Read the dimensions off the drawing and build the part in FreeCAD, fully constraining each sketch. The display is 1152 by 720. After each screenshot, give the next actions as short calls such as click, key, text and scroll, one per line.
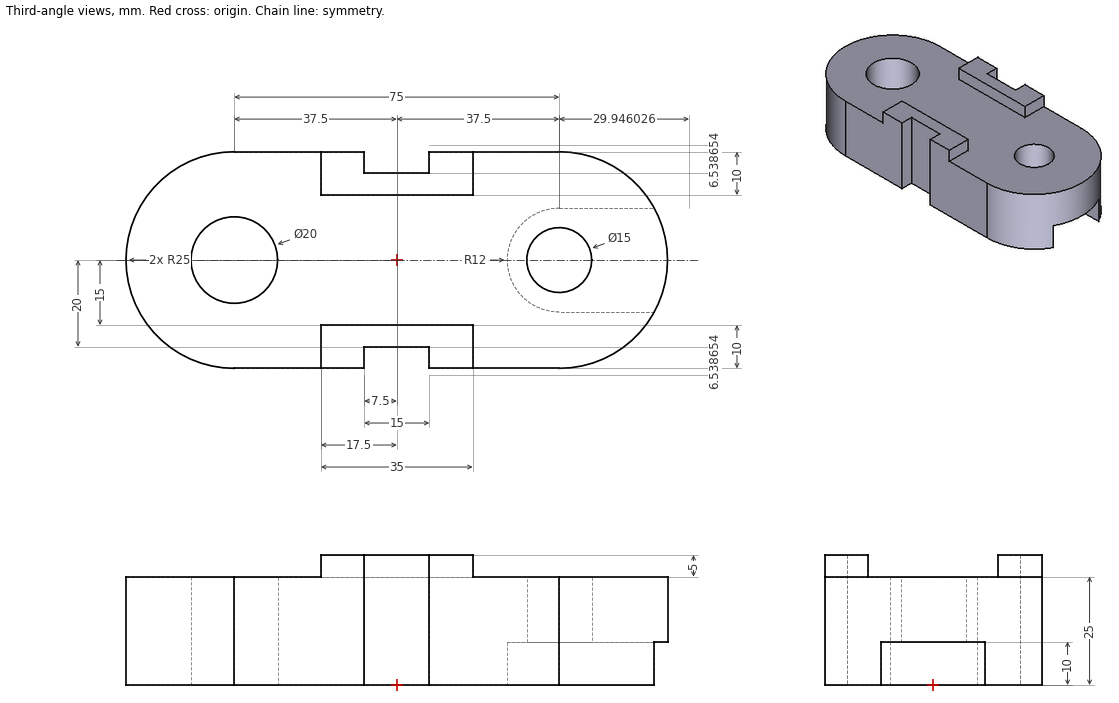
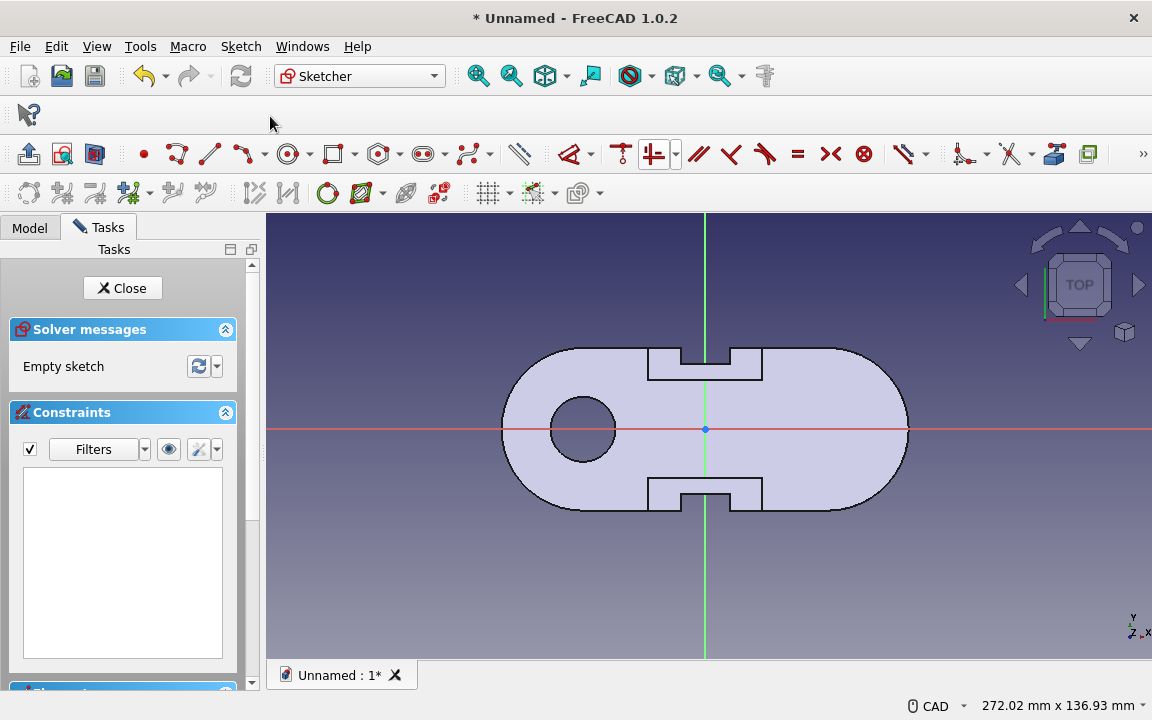
key(q)
key(s)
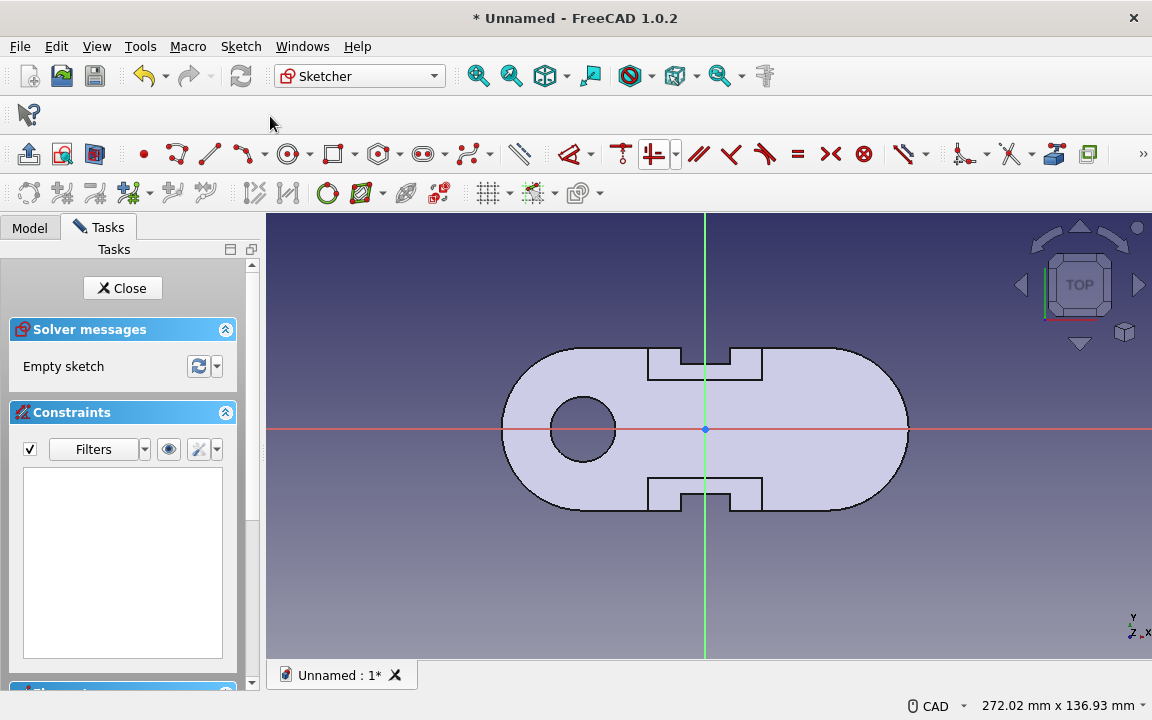
scroll(864, 428, up, 9)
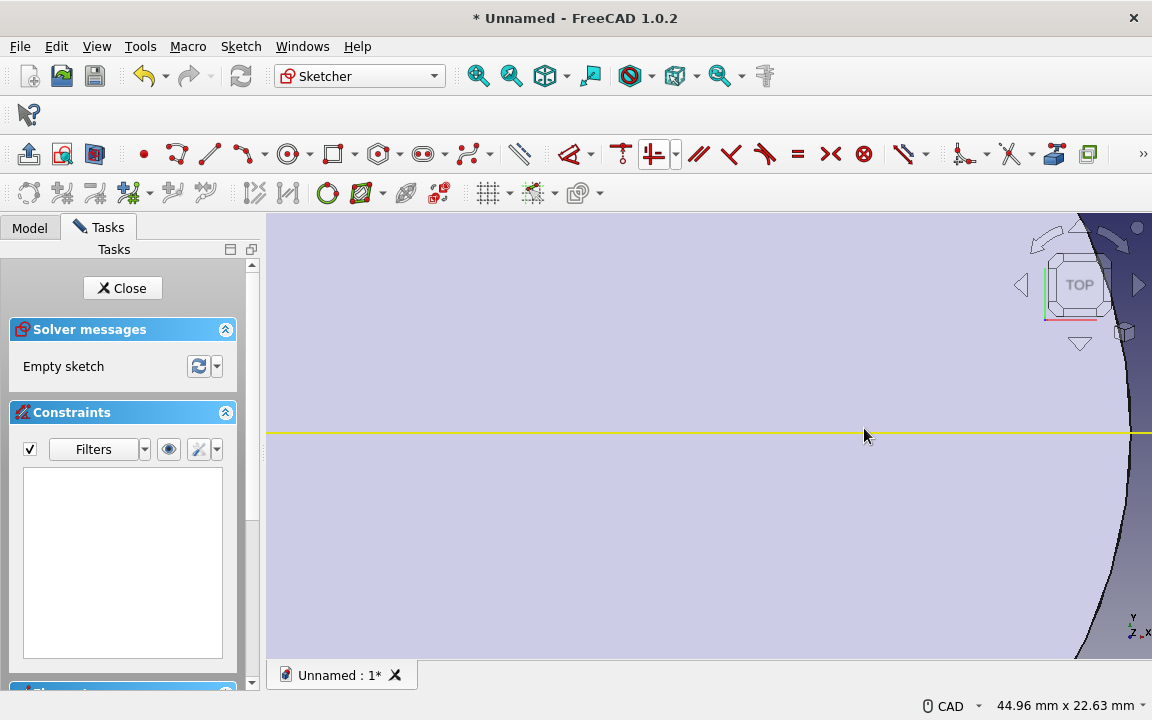
click(288, 154)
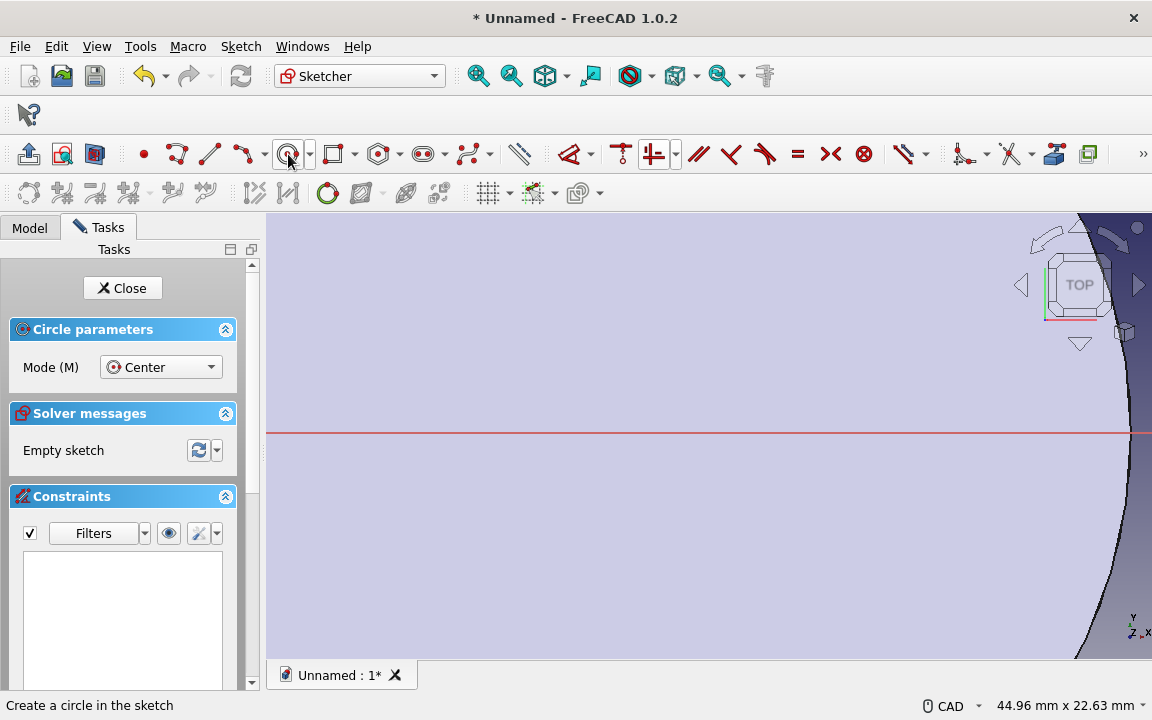
click(638, 433)
move(743, 329)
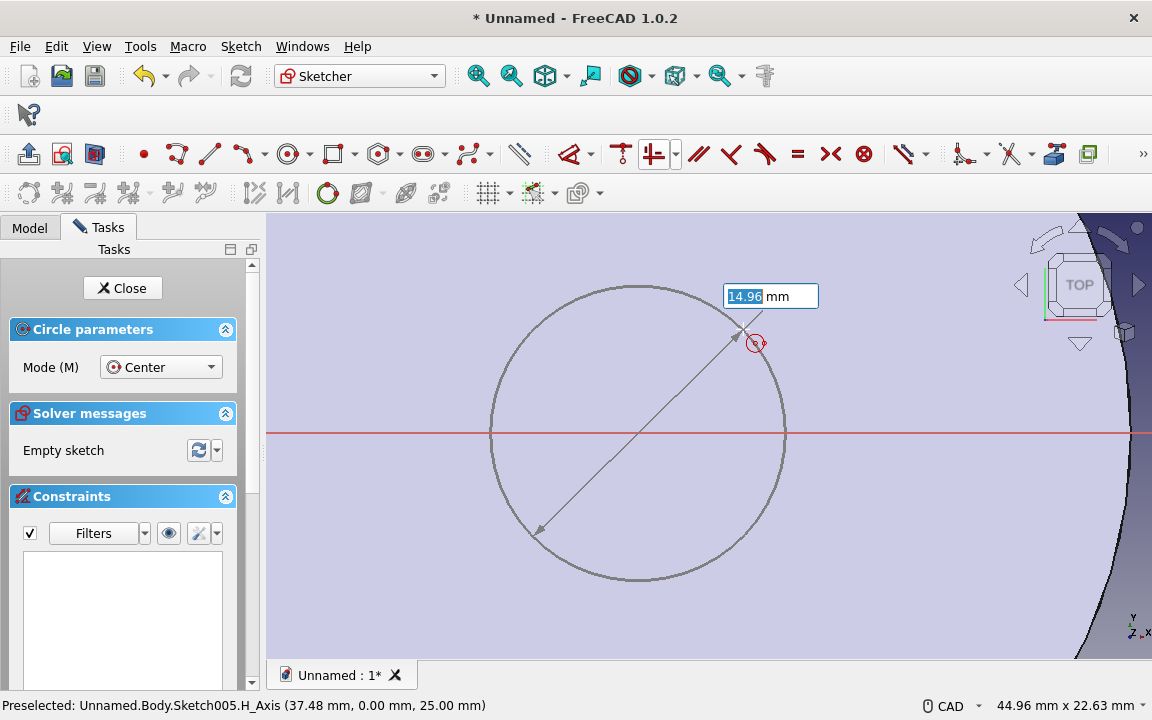
text(15)
key(Return)
key(Escape)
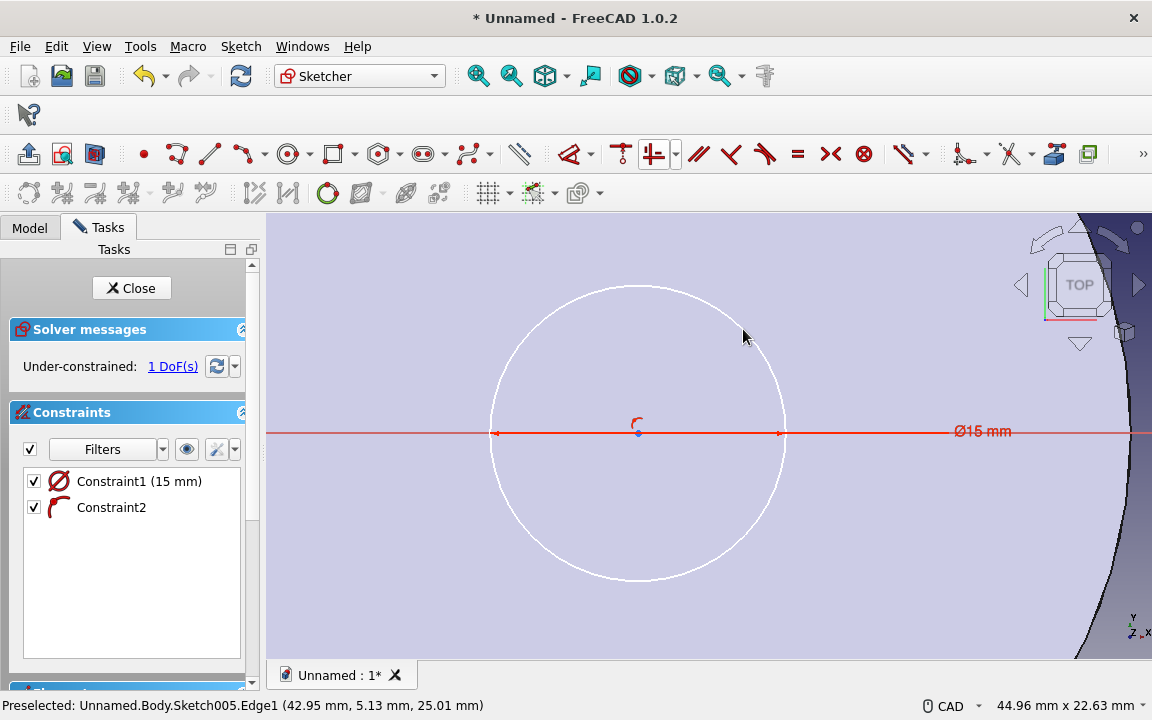
click(568, 154)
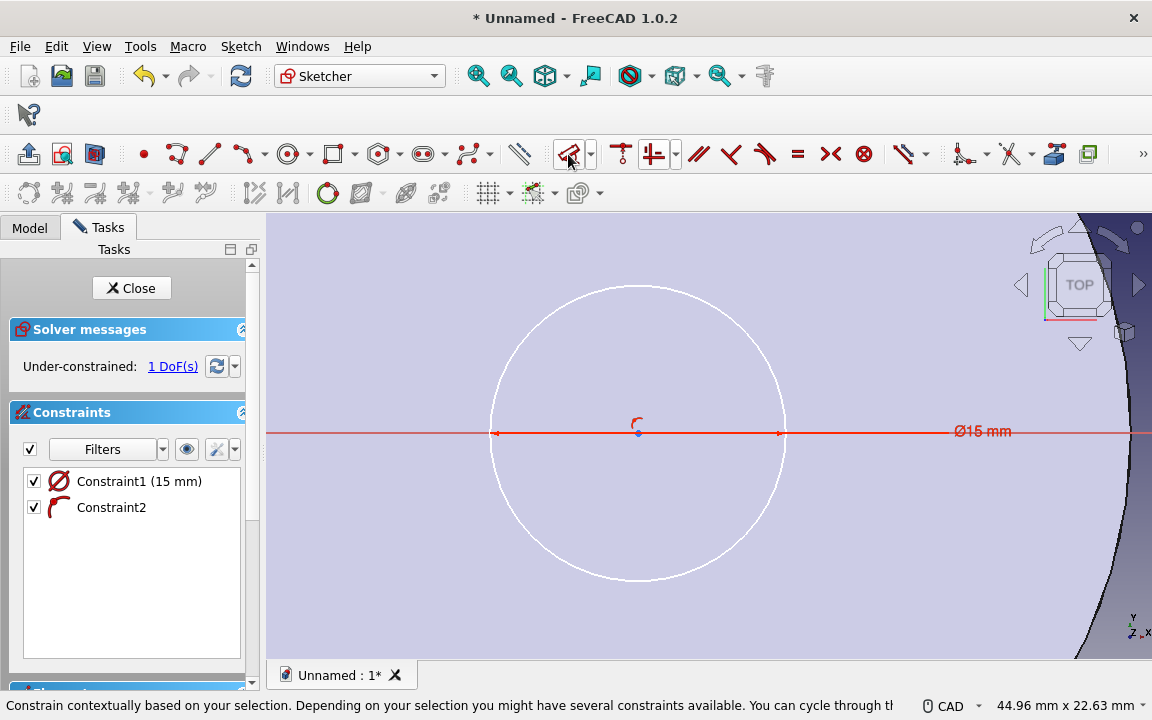
click(638, 433)
click(466, 467)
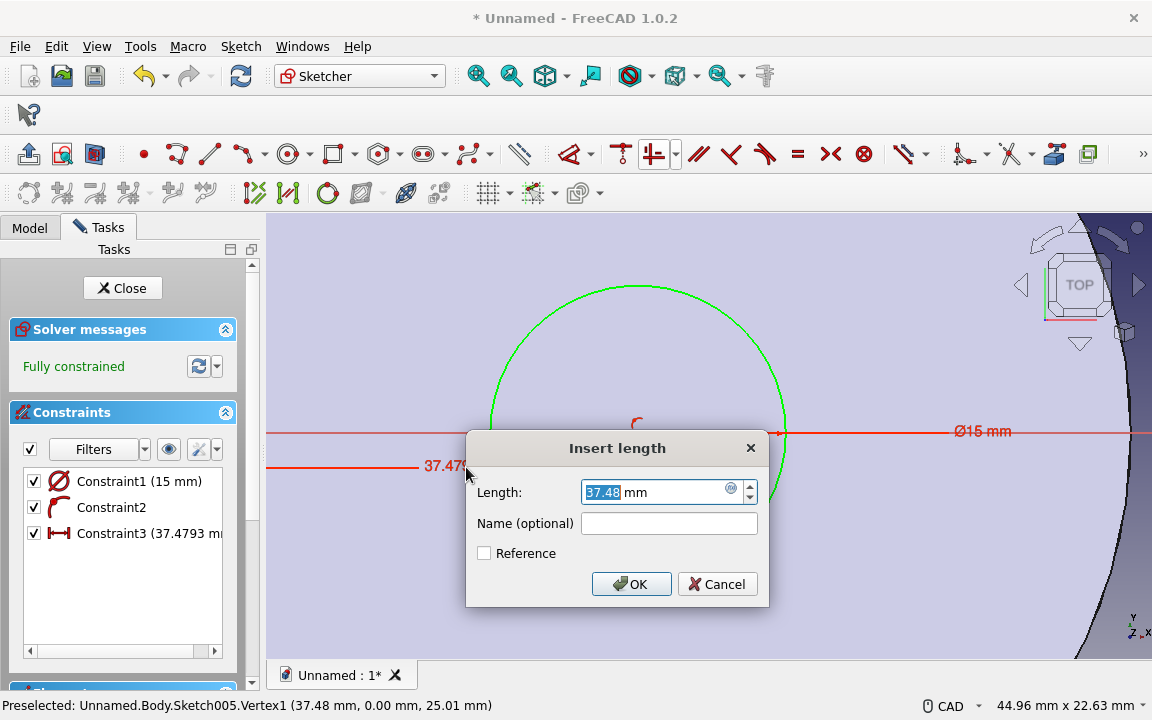
text(37.5)
key(Return)
key(Escape)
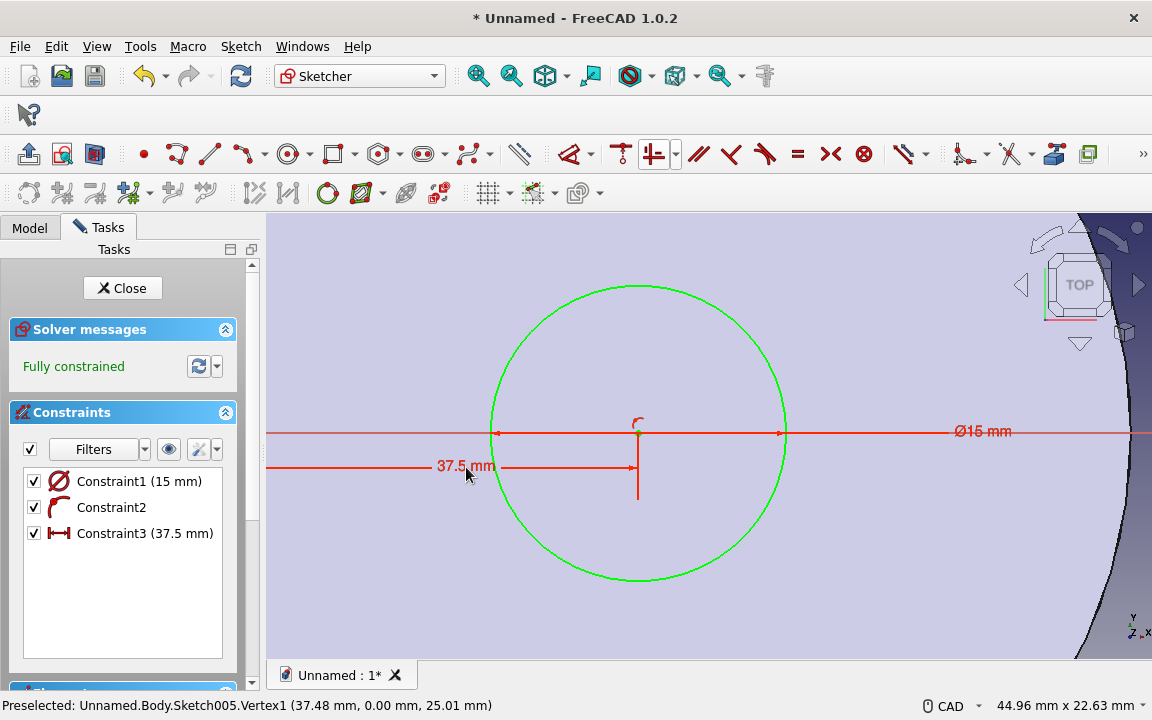
click(123, 288)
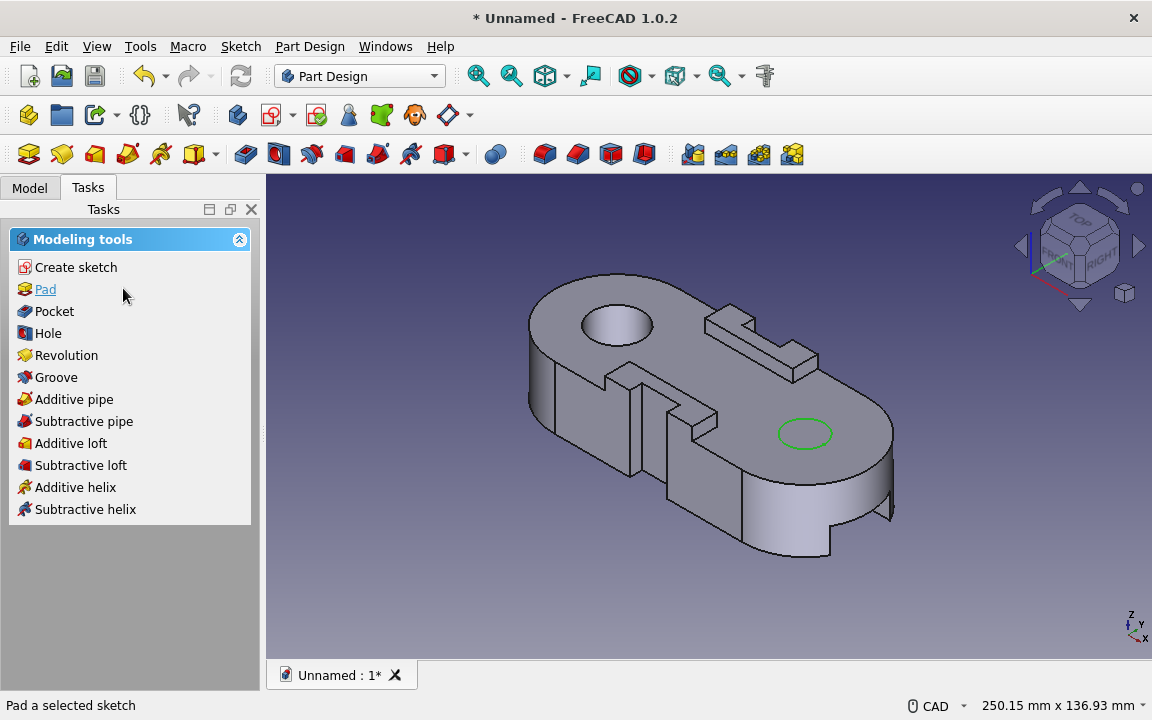
click(246, 154)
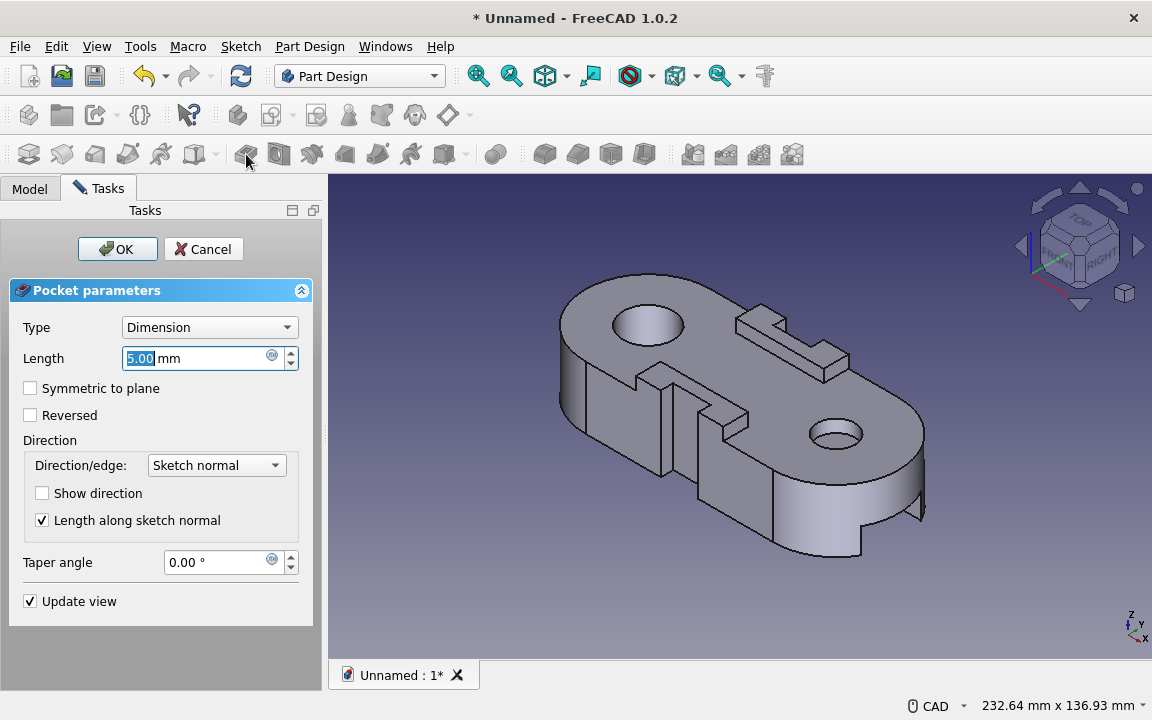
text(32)
key(Tab)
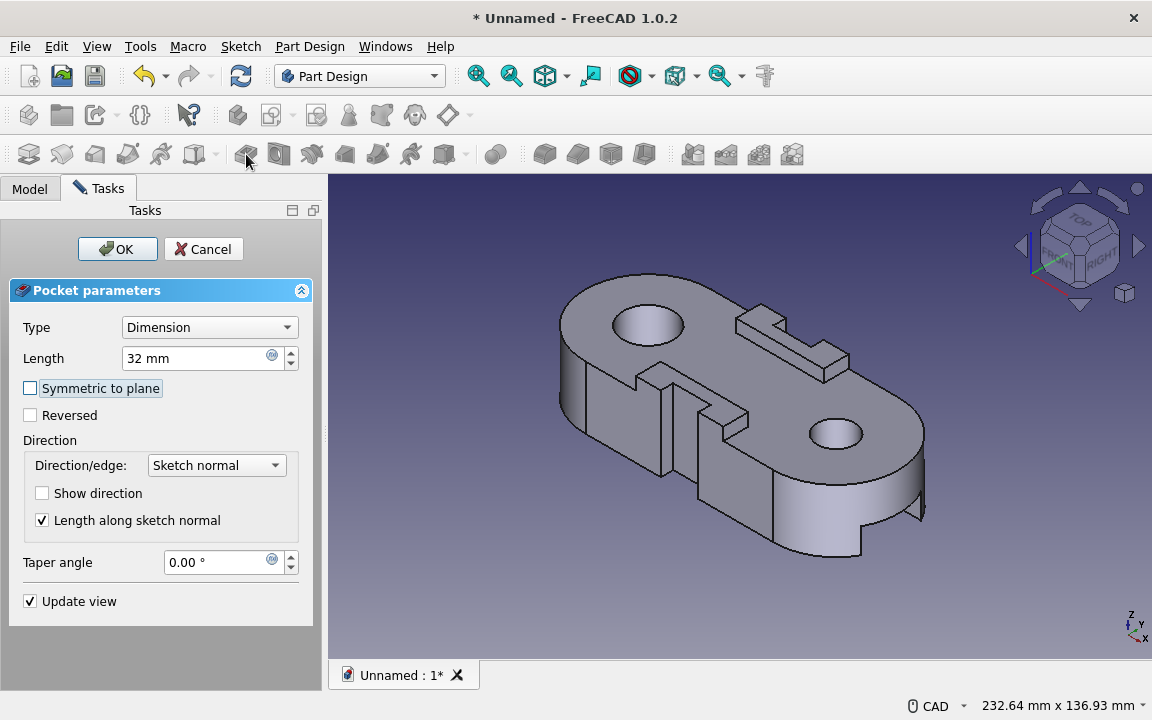
click(118, 249)